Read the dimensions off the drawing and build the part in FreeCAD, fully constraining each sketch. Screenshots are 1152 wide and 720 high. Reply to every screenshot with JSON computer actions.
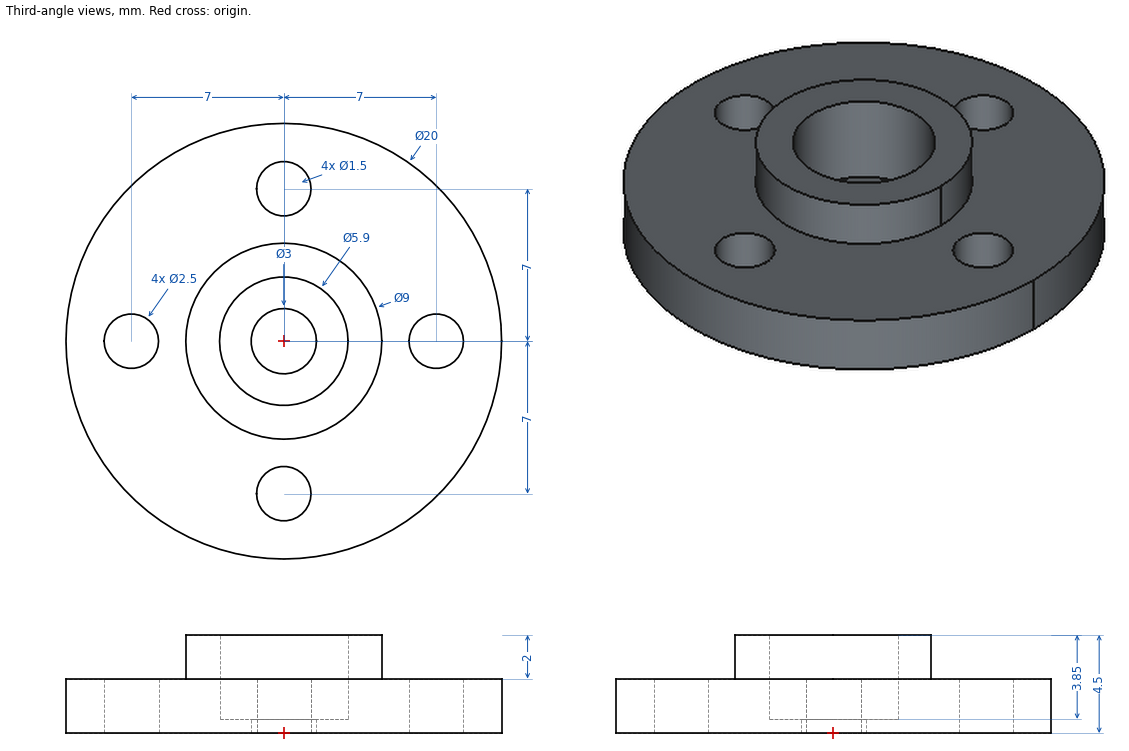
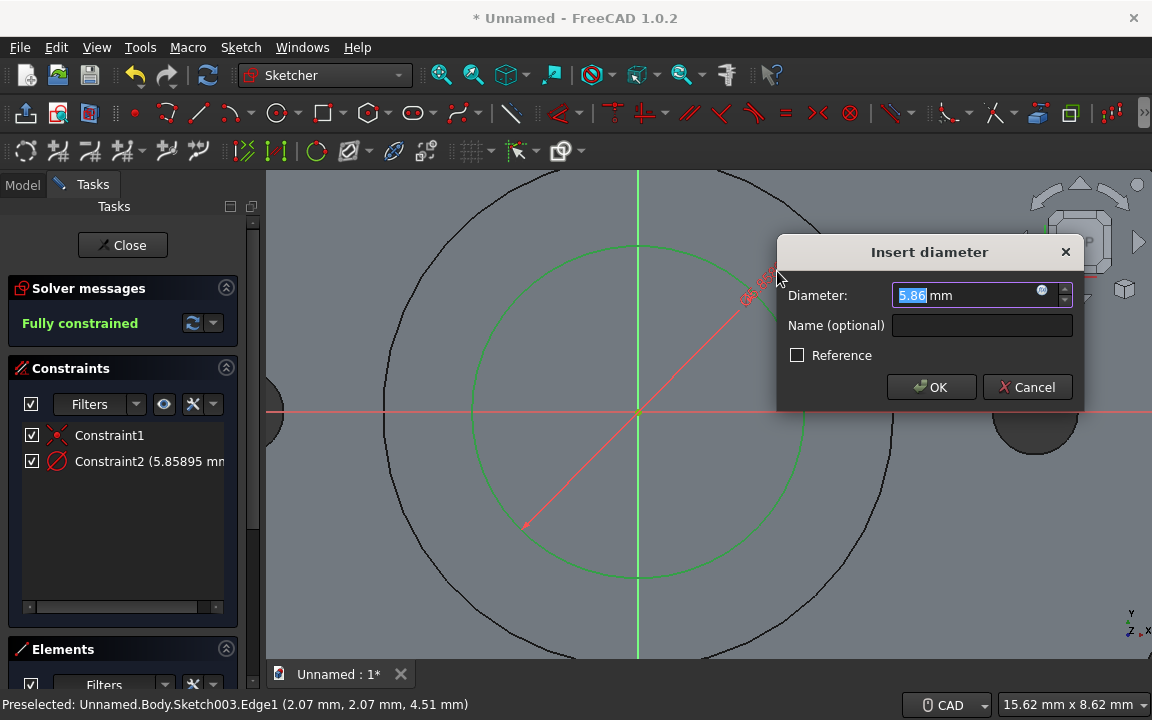
{"action": "type", "text": "5.9"}
{"action": "key", "text": "Return"}
{"action": "key", "text": "Escape"}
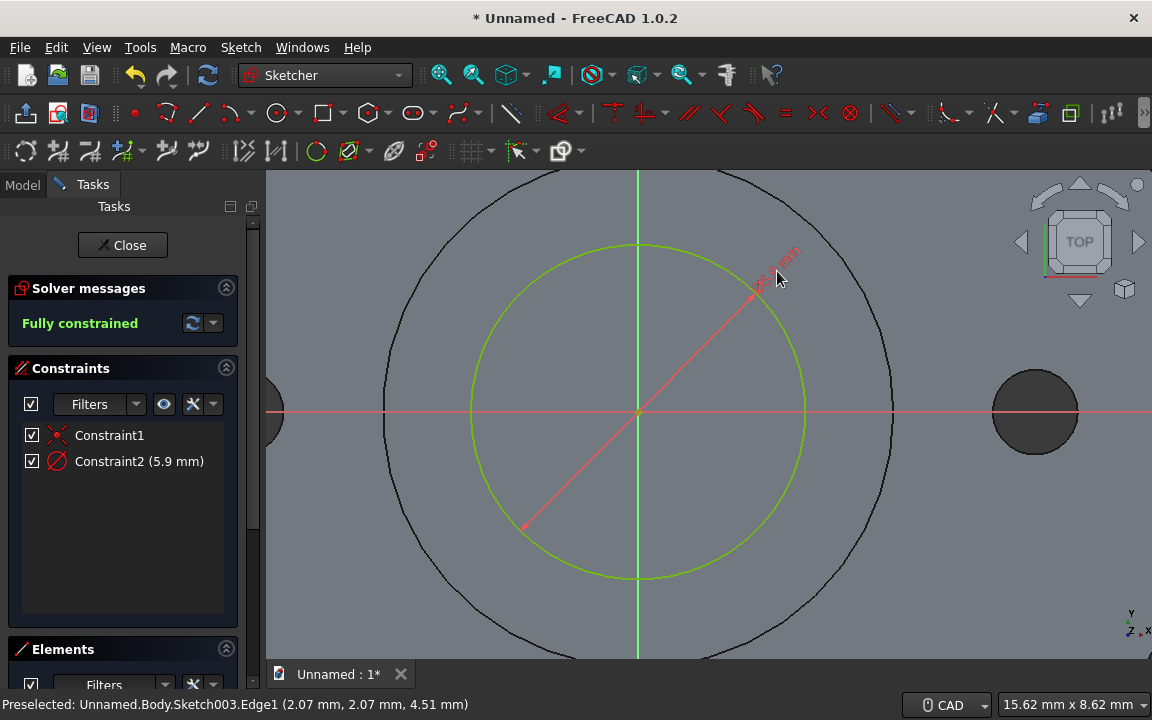
{"action": "left_click", "coordinate": [123, 245]}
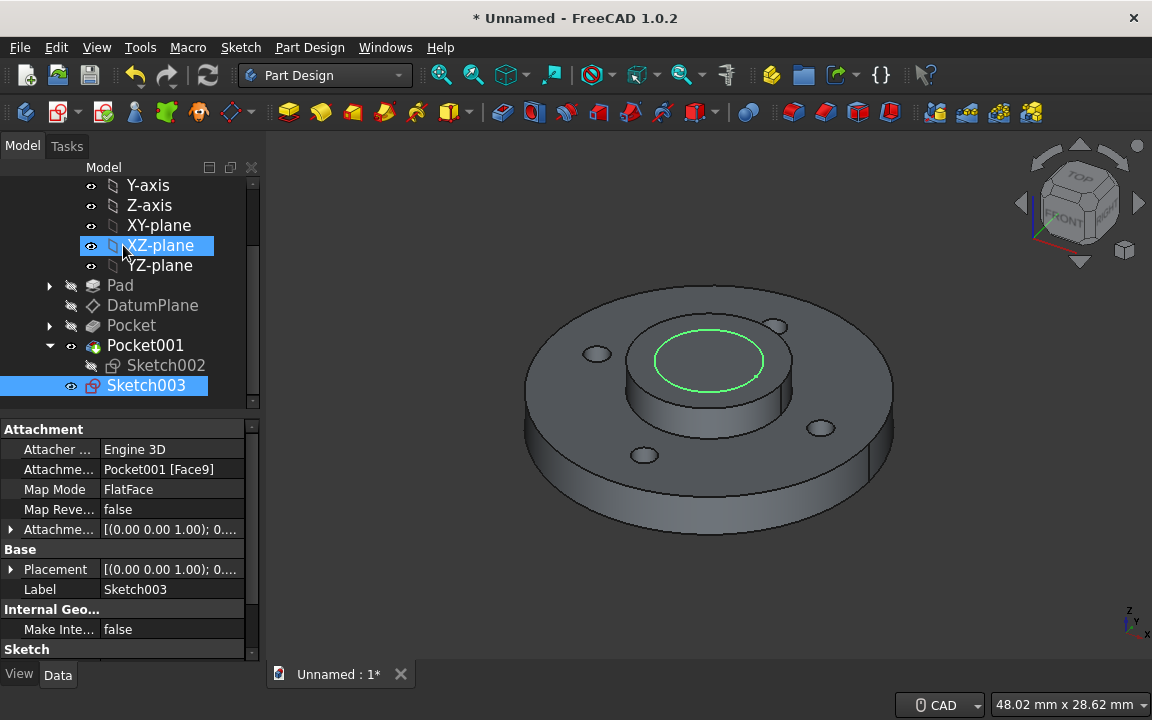
{"action": "left_click", "coordinate": [504, 112]}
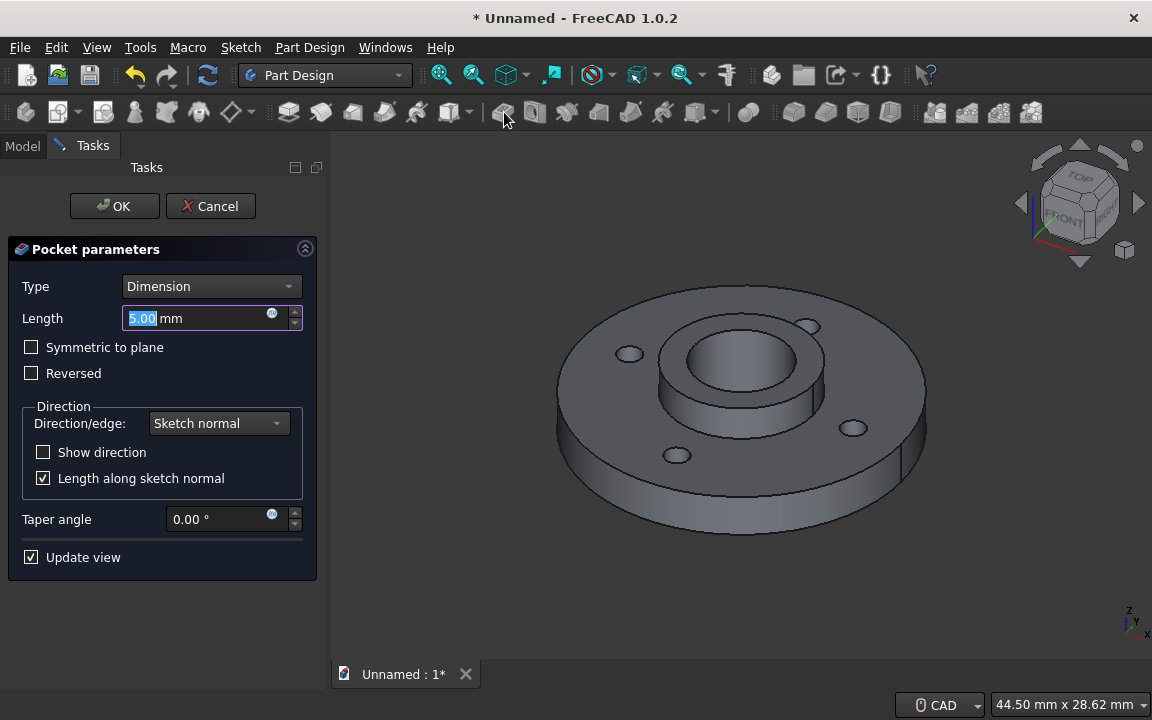
{"action": "type", "text": "3.85"}
{"action": "key", "text": "Tab"}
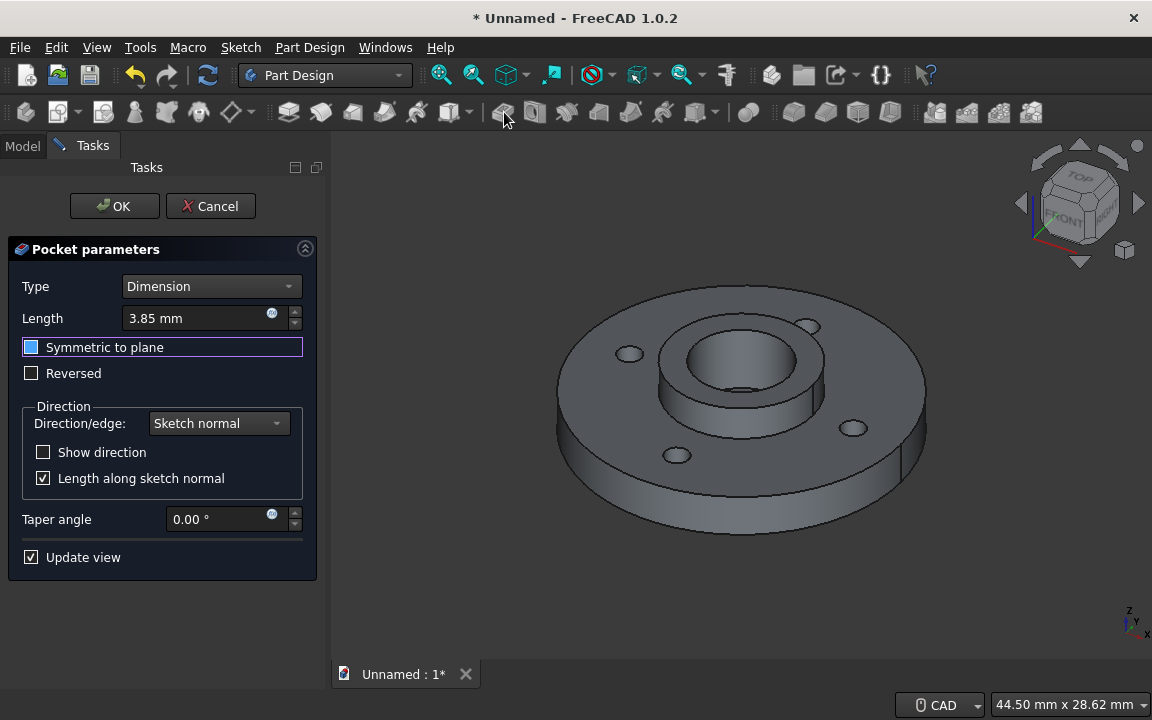
{"action": "left_click", "coordinate": [115, 206]}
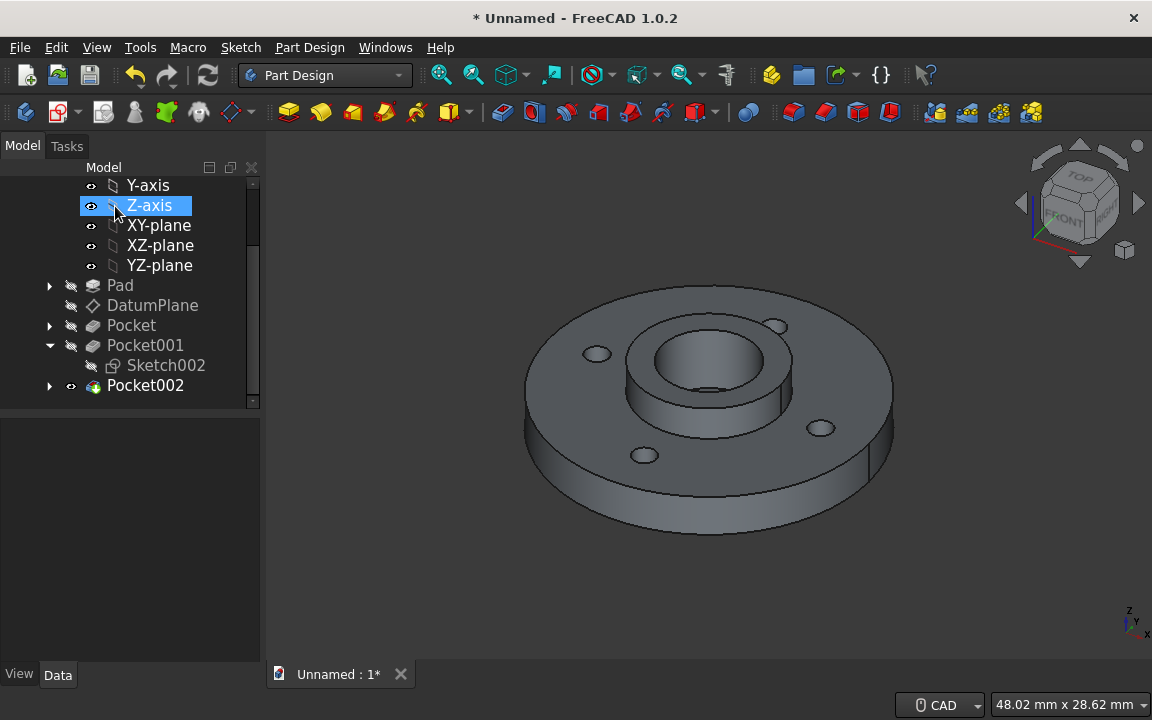
{"action": "key", "text": "0"}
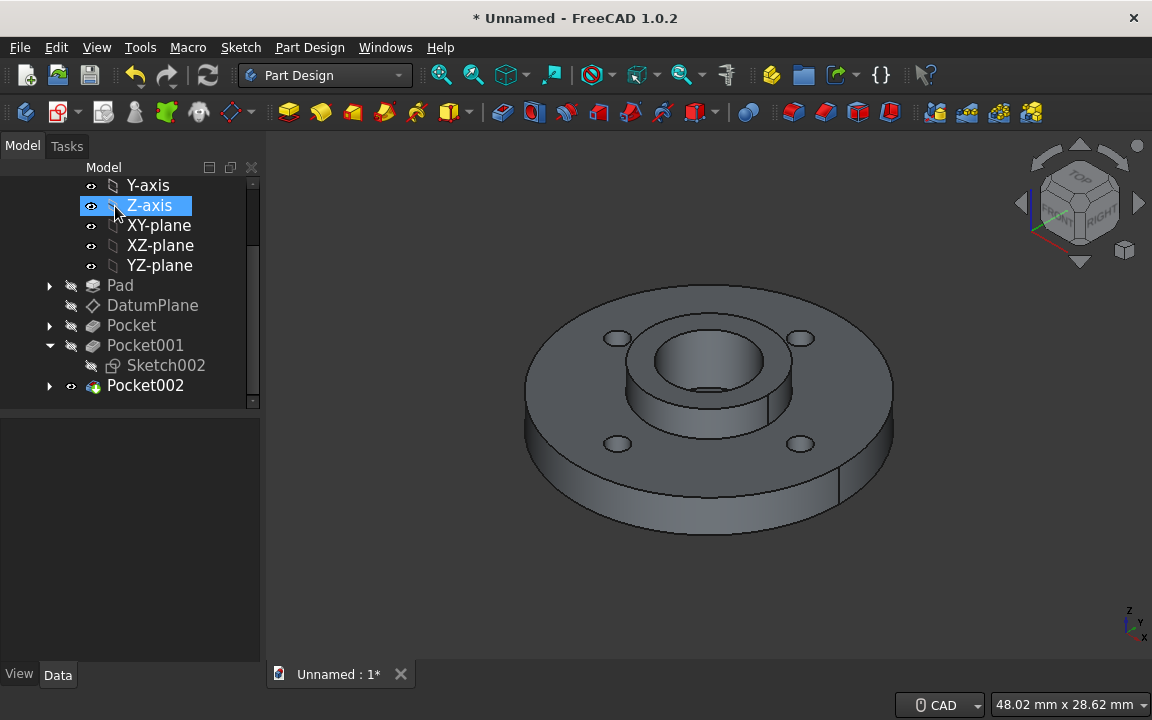
{"action": "key", "text": "2"}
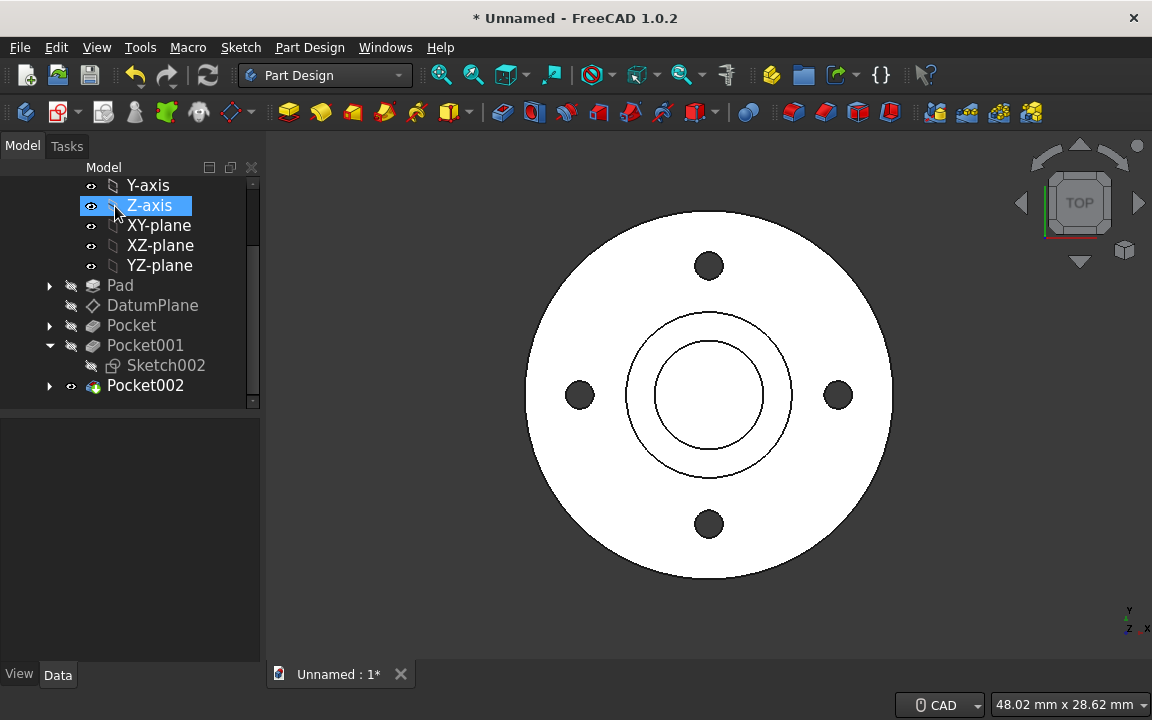
{"action": "left_click", "coordinate": [709, 394]}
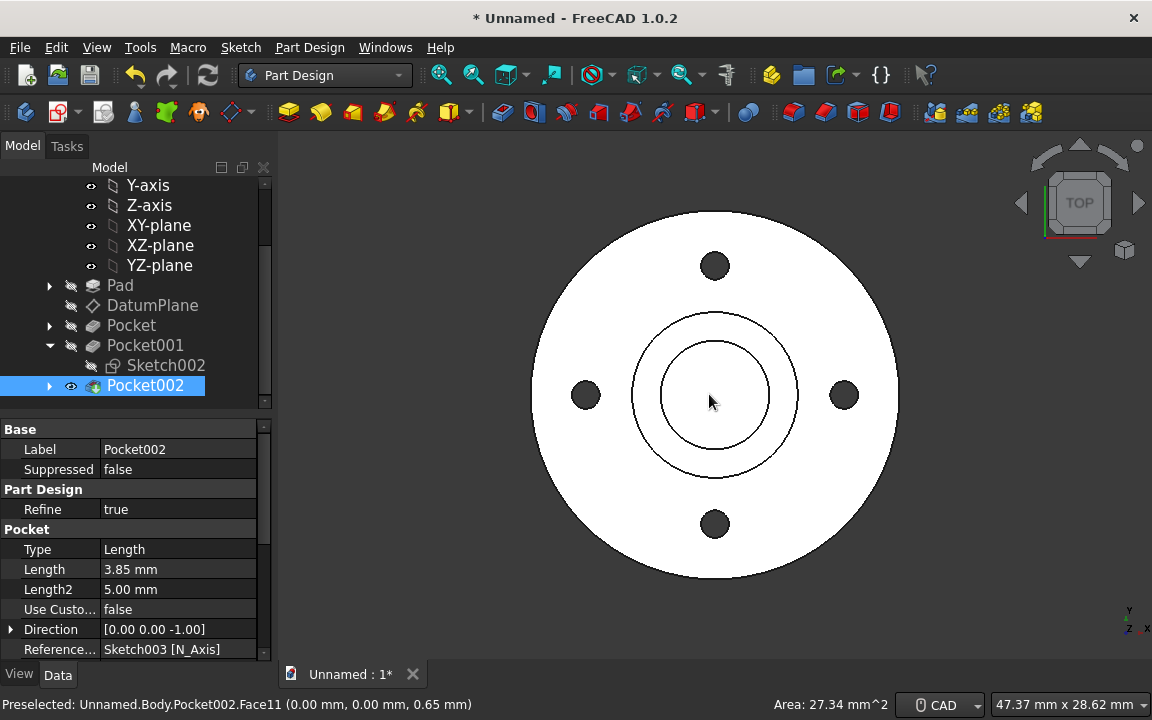
{"action": "left_click", "coordinate": [58, 112]}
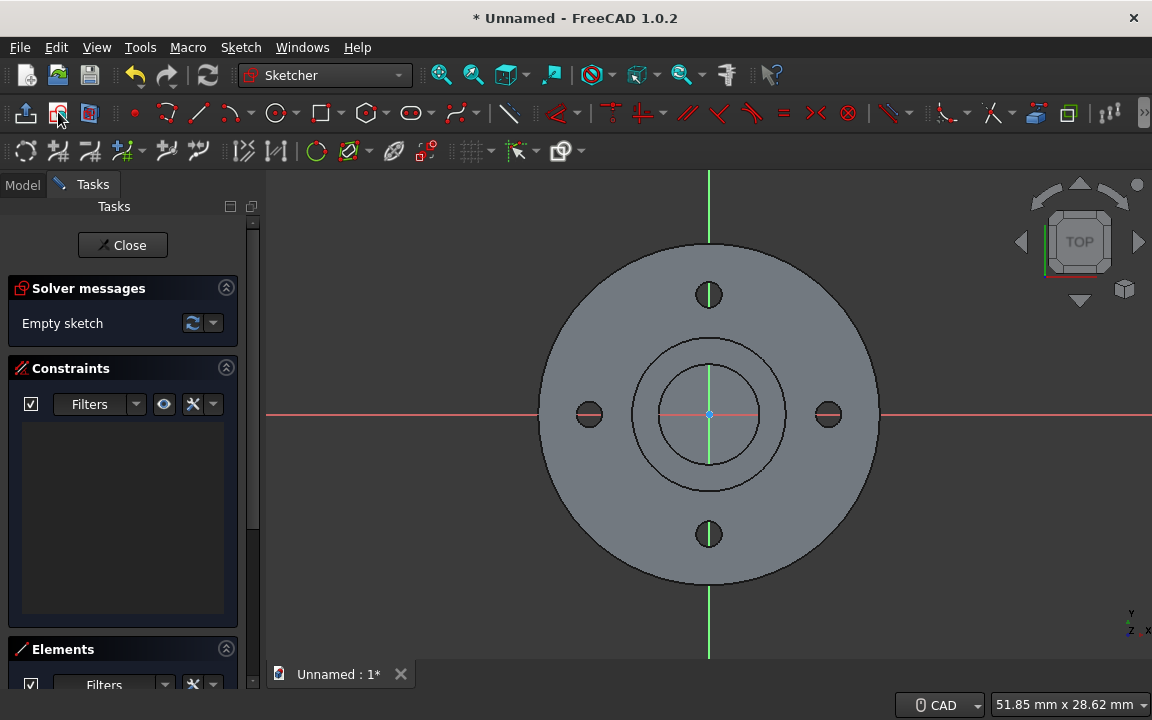
{"action": "key", "text": "q s"}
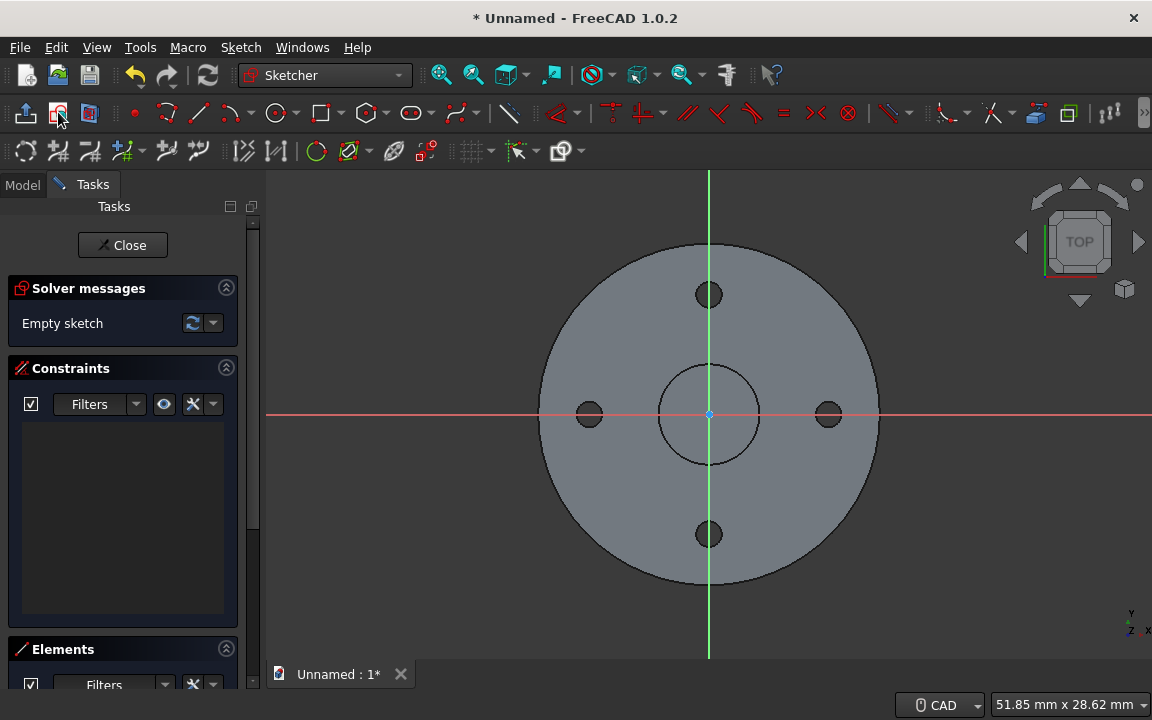
{"action": "scroll", "coordinate": [723, 414], "scroll_direction": "up", "scroll_amount": 9}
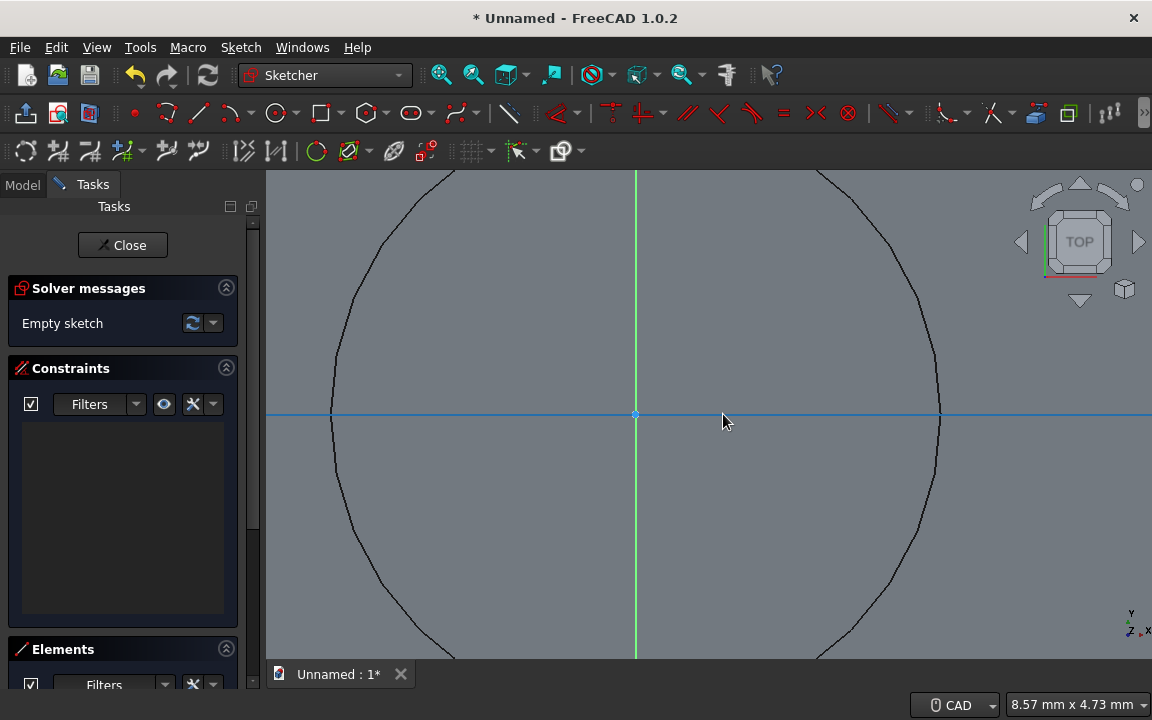
{"action": "key", "text": "g c"}